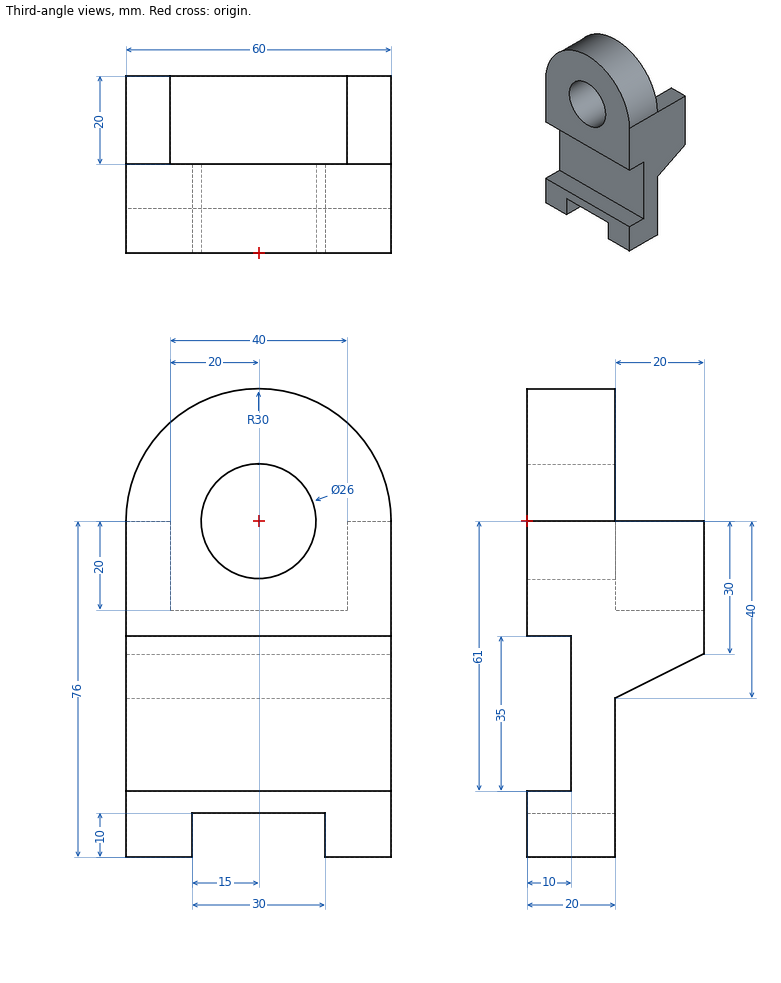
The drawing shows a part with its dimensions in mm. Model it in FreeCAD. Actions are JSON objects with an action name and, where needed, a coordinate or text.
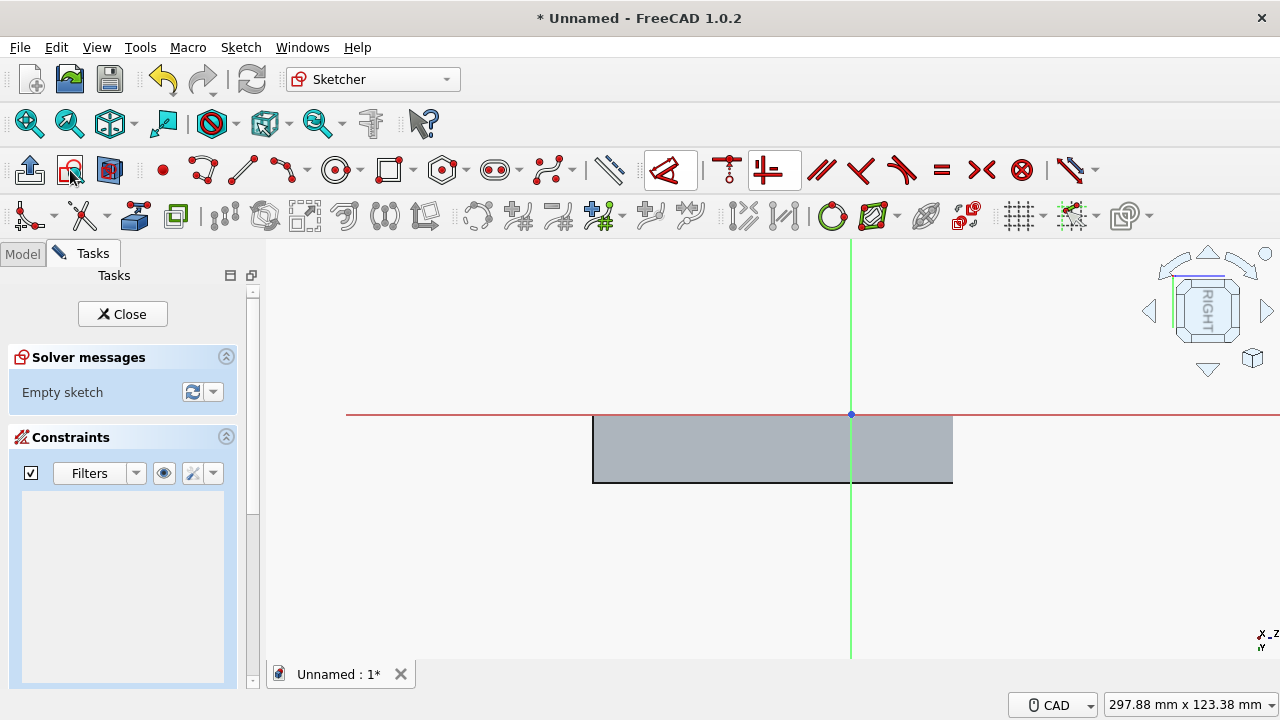
{"action": "scroll", "coordinate": [773, 422], "scroll_direction": "up", "scroll_amount": 5}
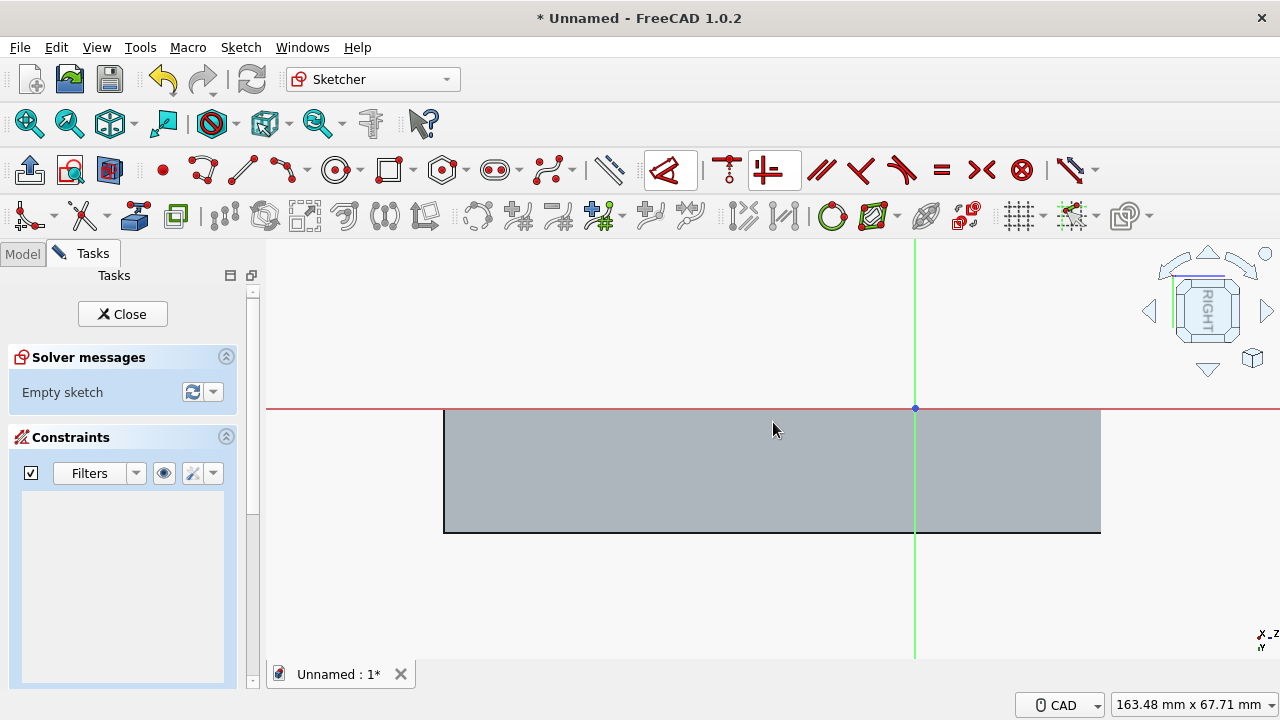
{"action": "key", "text": "g r"}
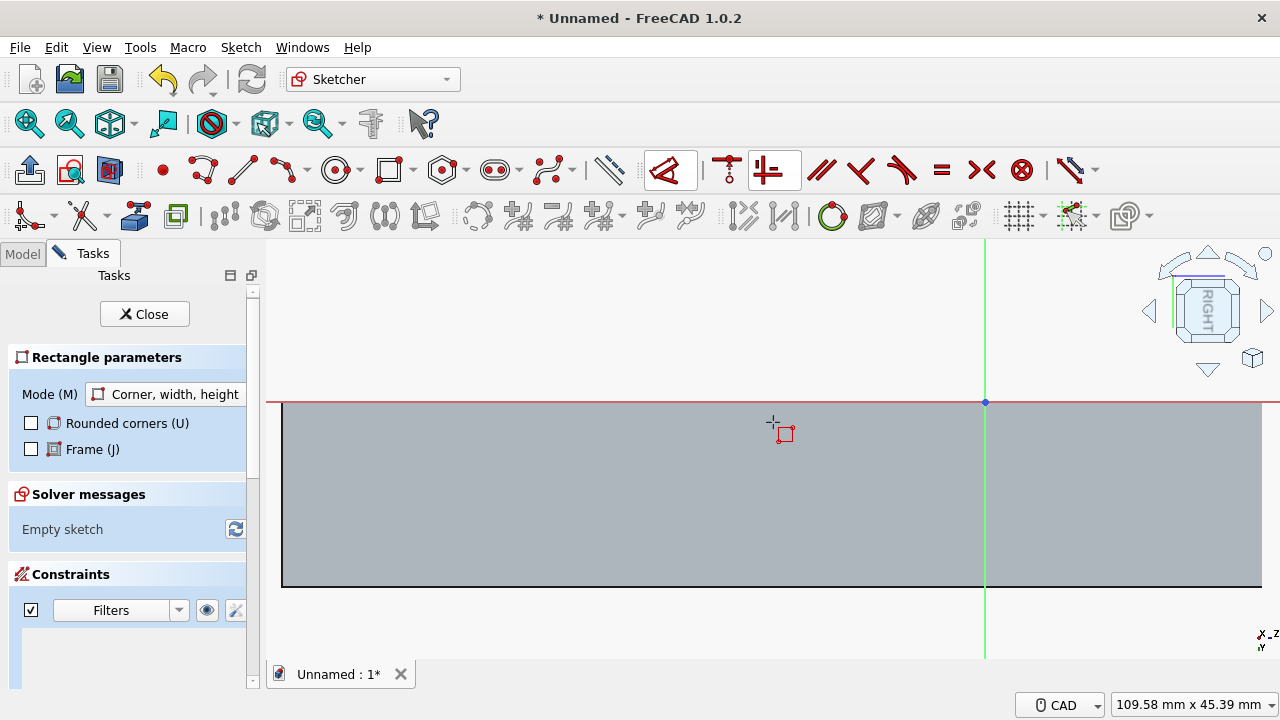
{"action": "left_click", "coordinate": [421, 402]}
{"action": "left_click", "coordinate": [745, 495]}
{"action": "key", "text": "Escape"}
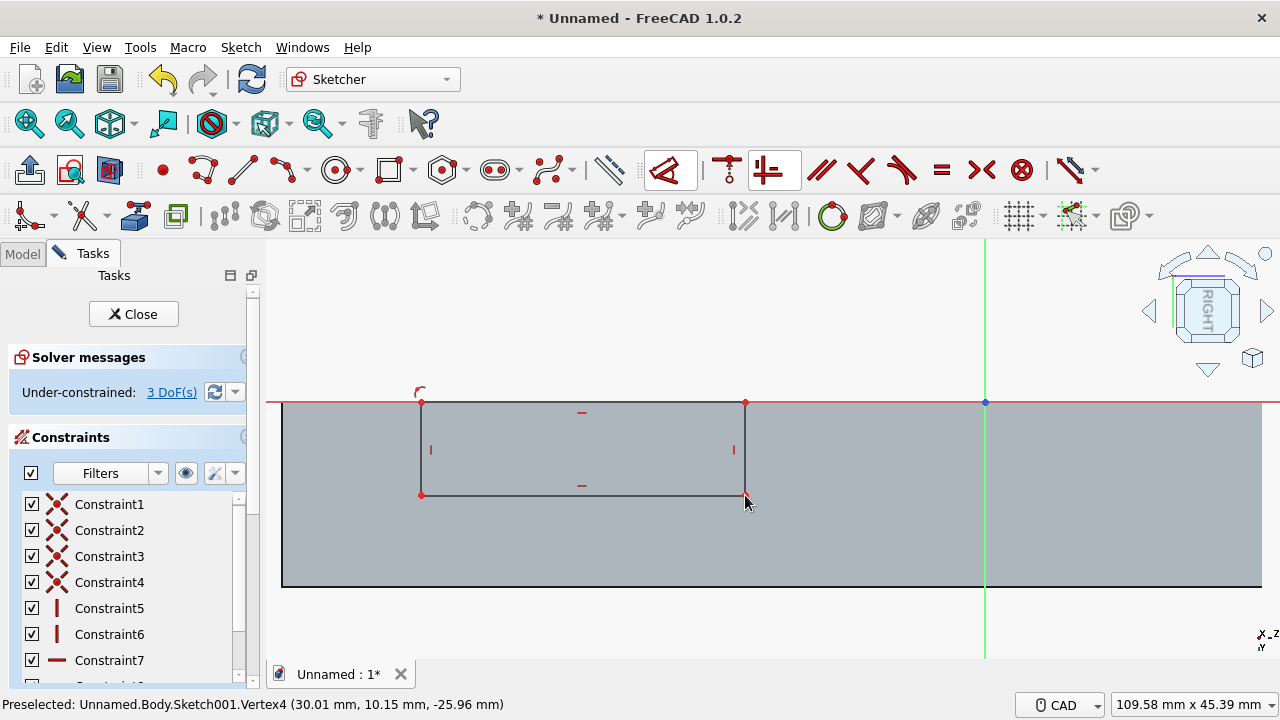
{"action": "left_click", "coordinate": [421, 430]}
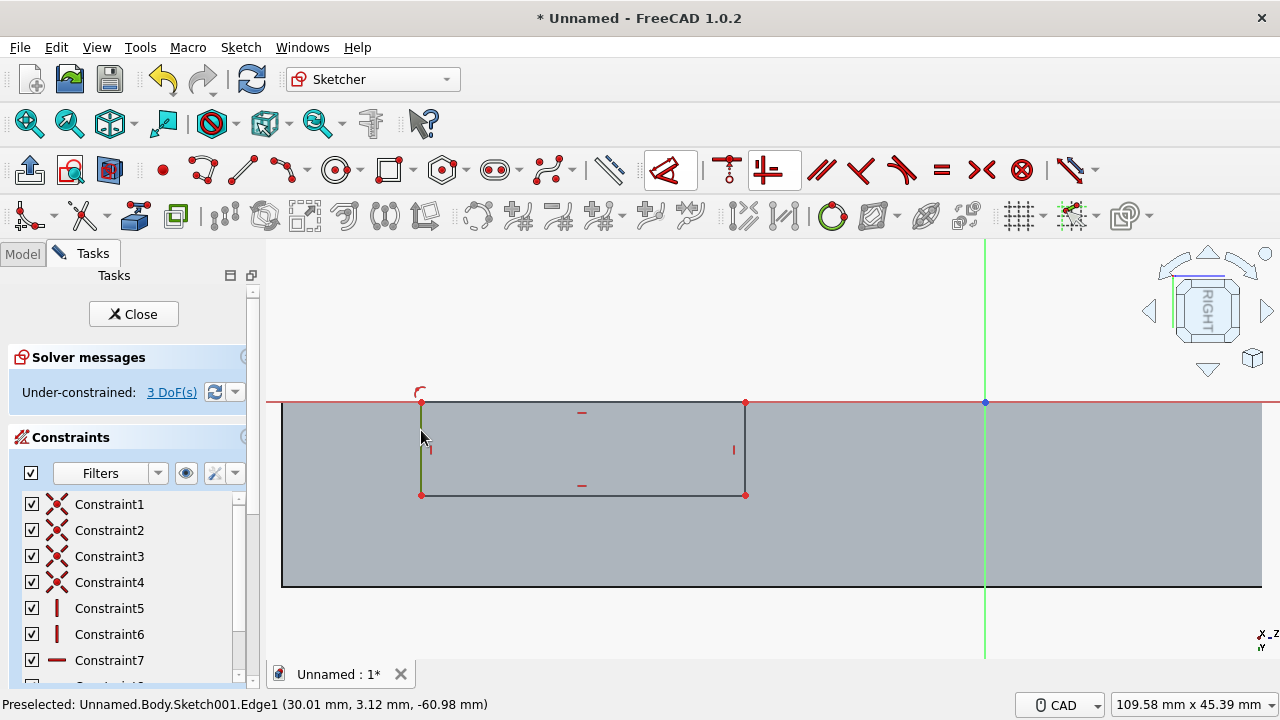
{"action": "key", "text": "i"}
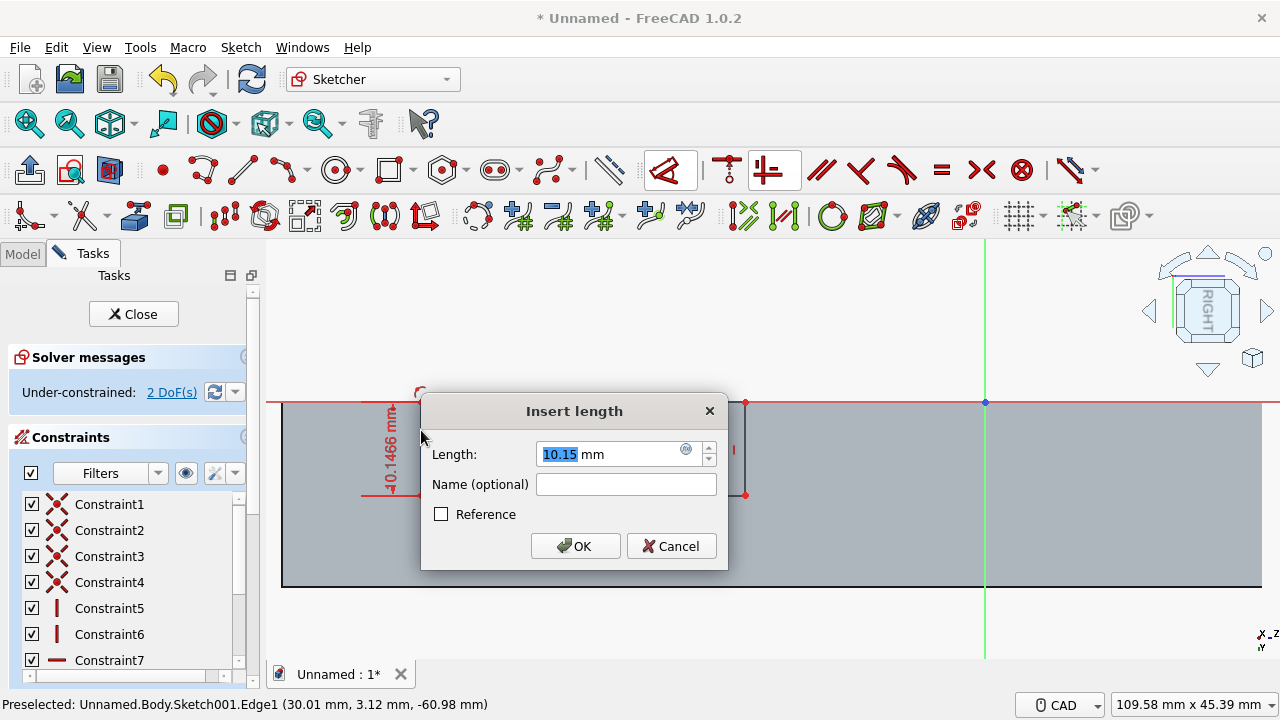
{"action": "type", "text": "10"}
{"action": "key", "text": "Return"}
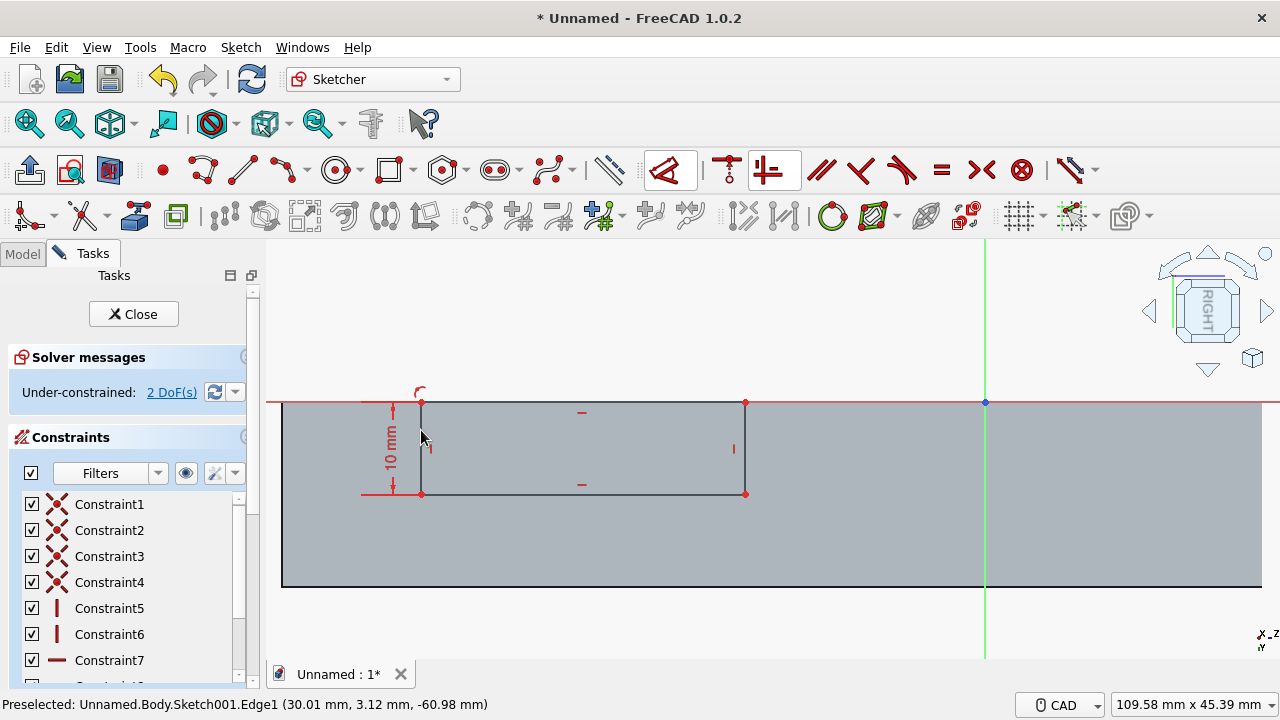
{"action": "left_click", "coordinate": [518, 495]}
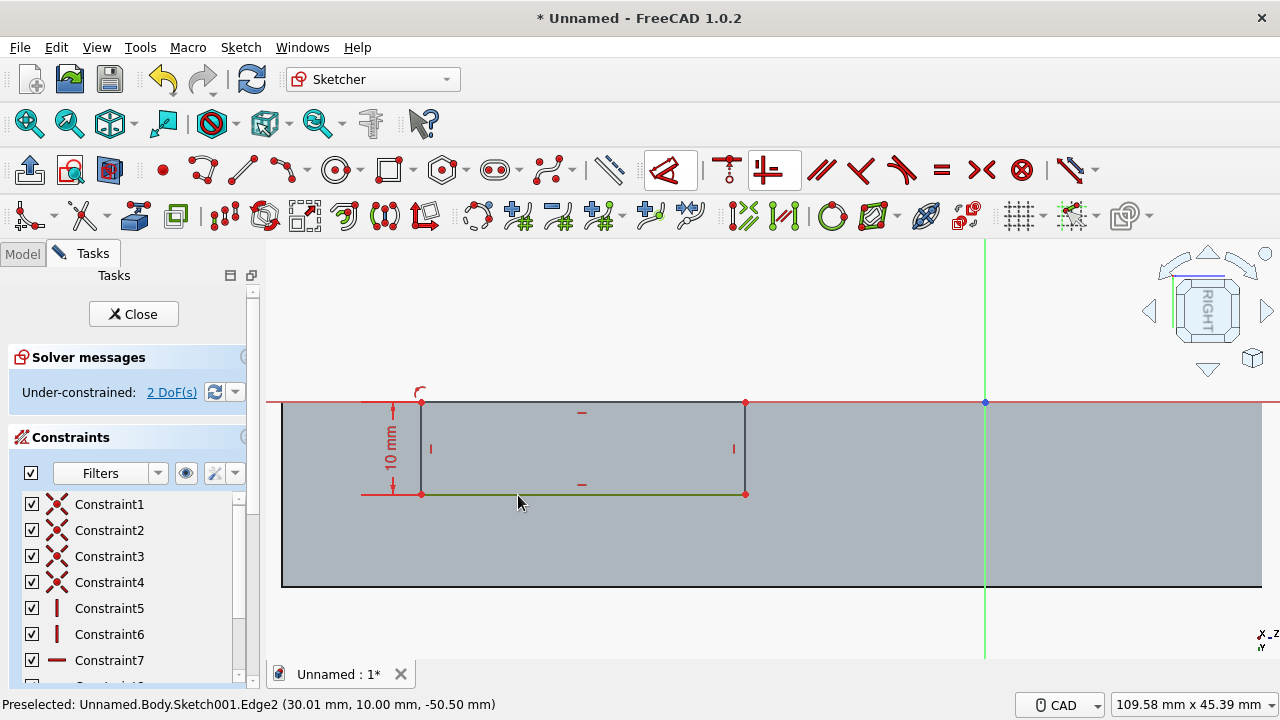
{"action": "key", "text": "l"}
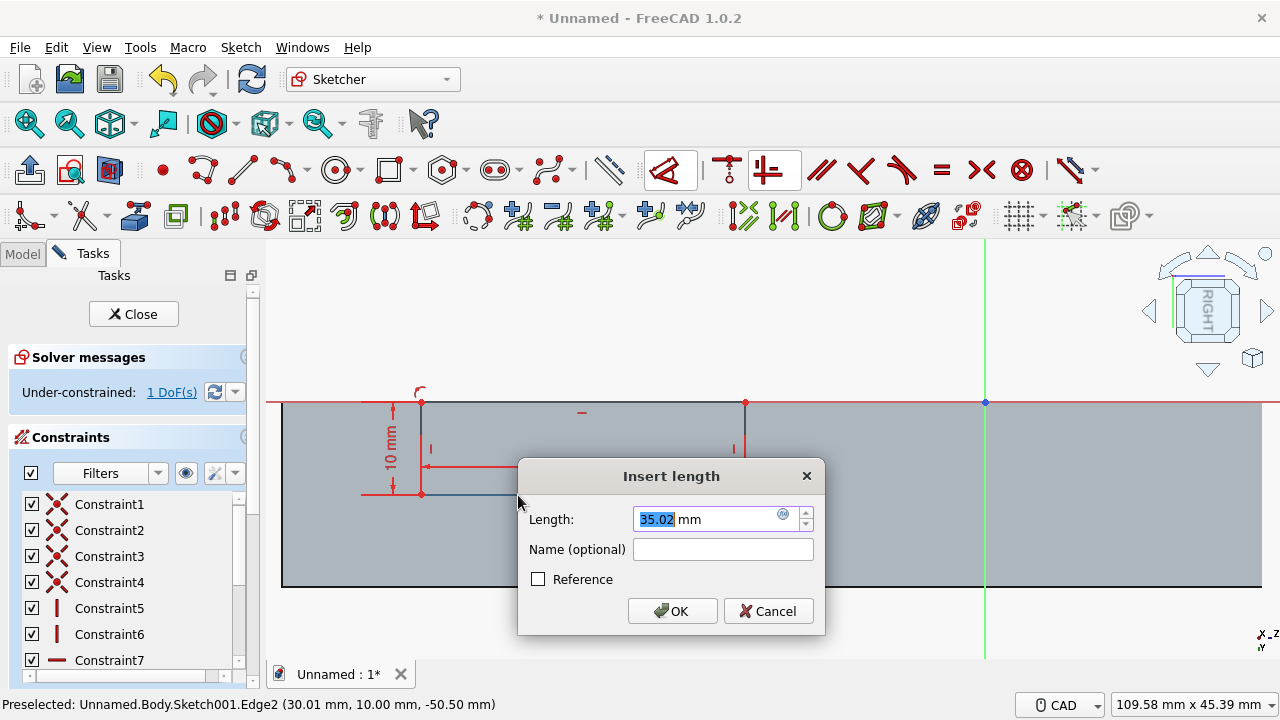
{"action": "type", "text": "35"}
{"action": "key", "text": "Return"}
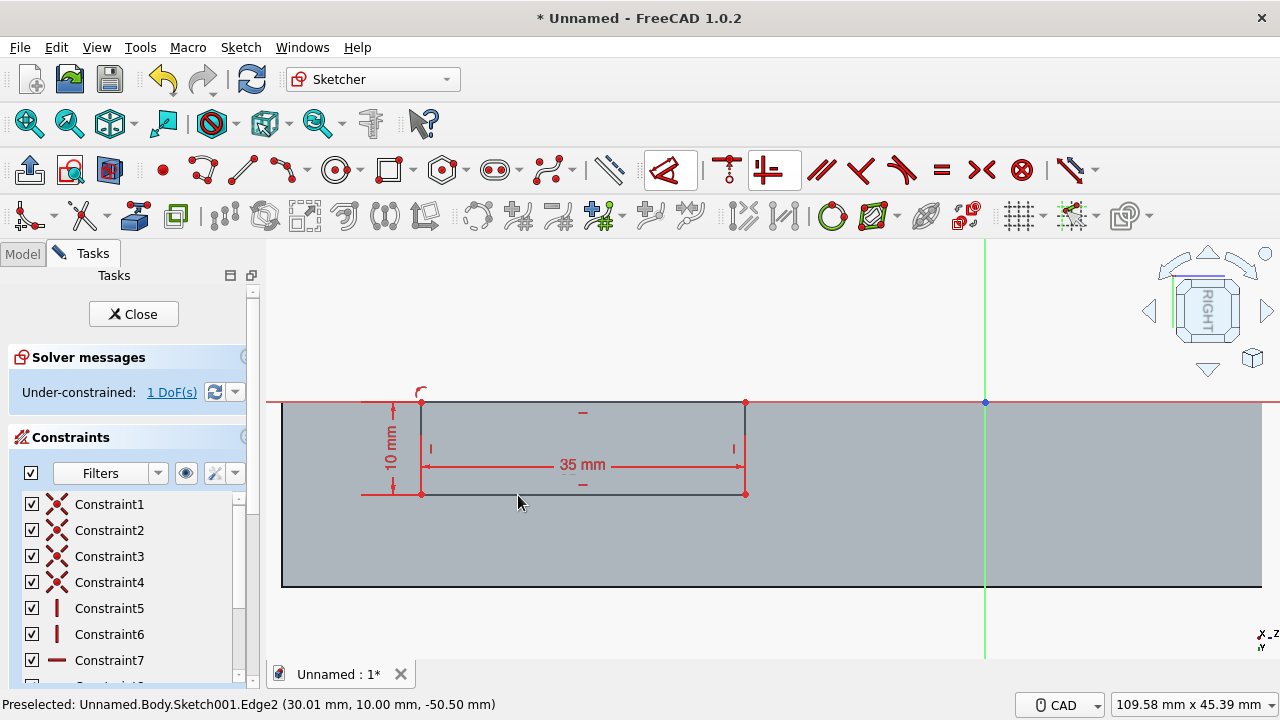
{"action": "left_click", "coordinate": [421, 402]}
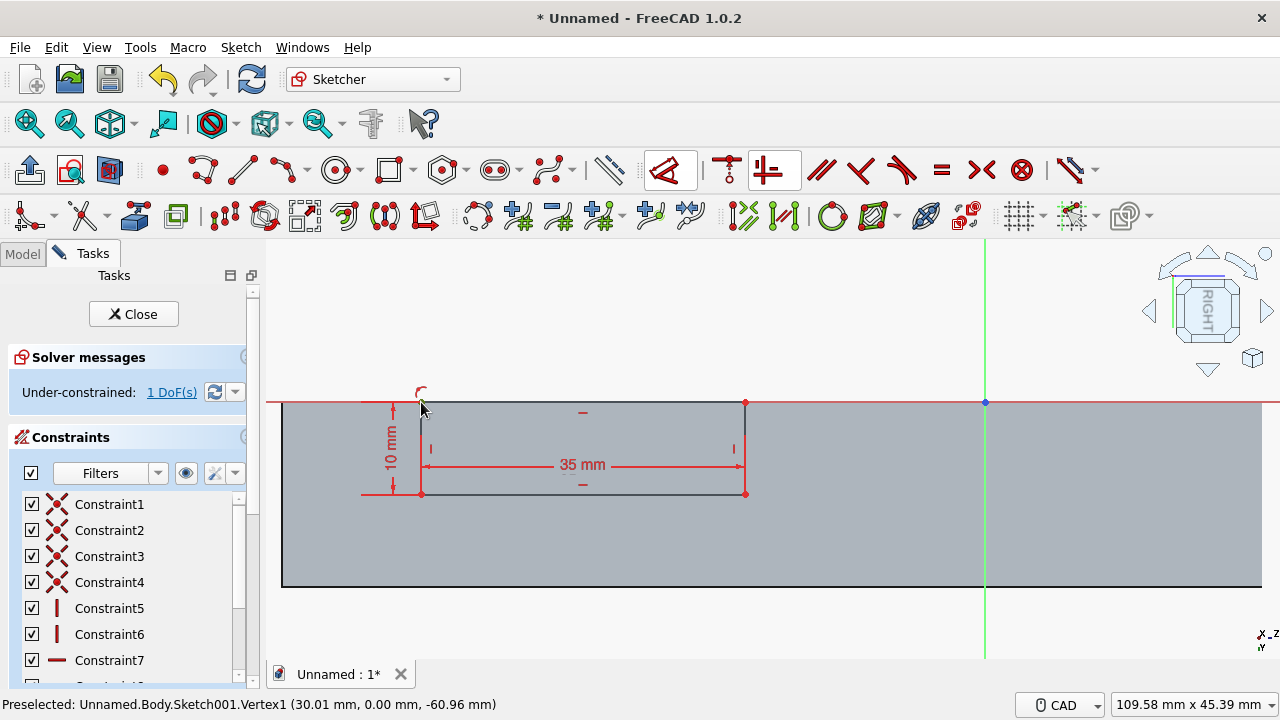
{"action": "left_click", "coordinate": [692, 170]}